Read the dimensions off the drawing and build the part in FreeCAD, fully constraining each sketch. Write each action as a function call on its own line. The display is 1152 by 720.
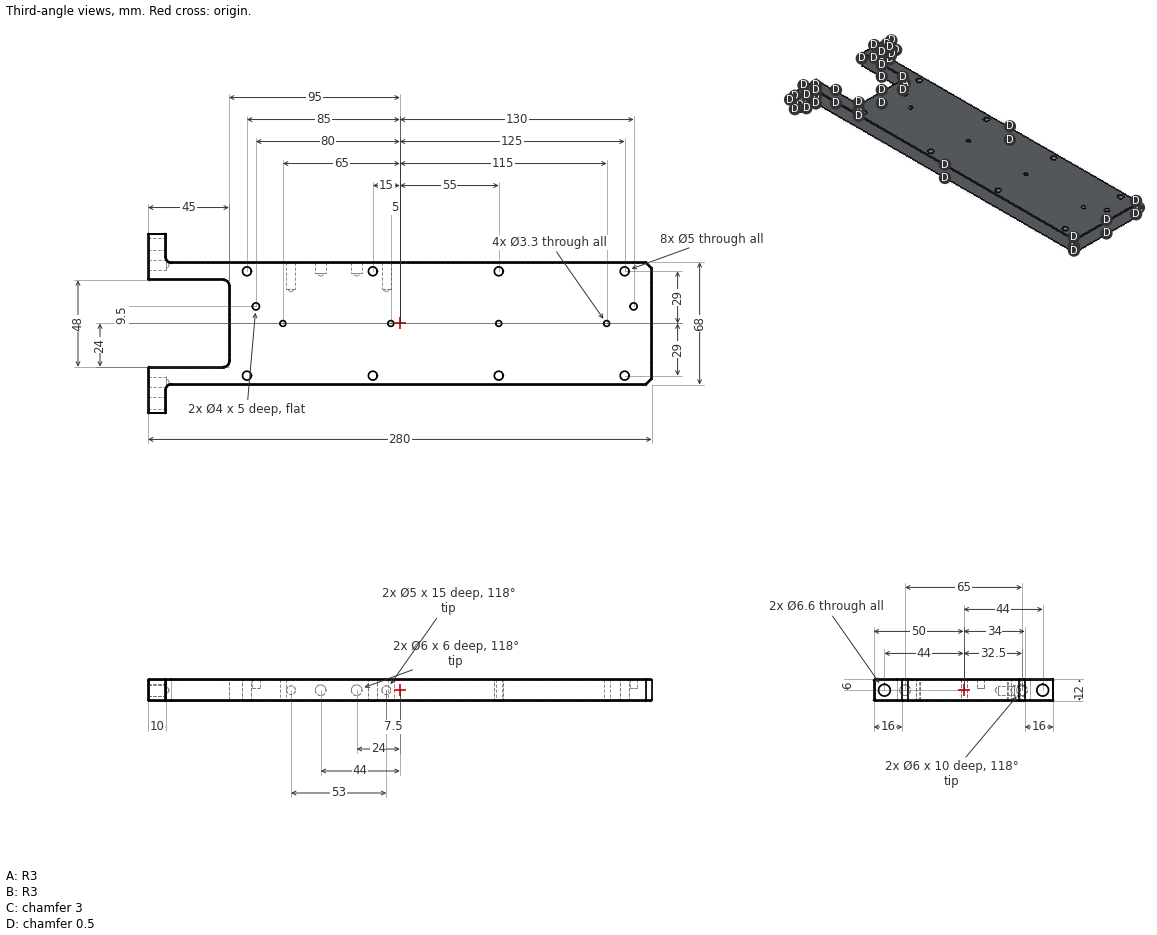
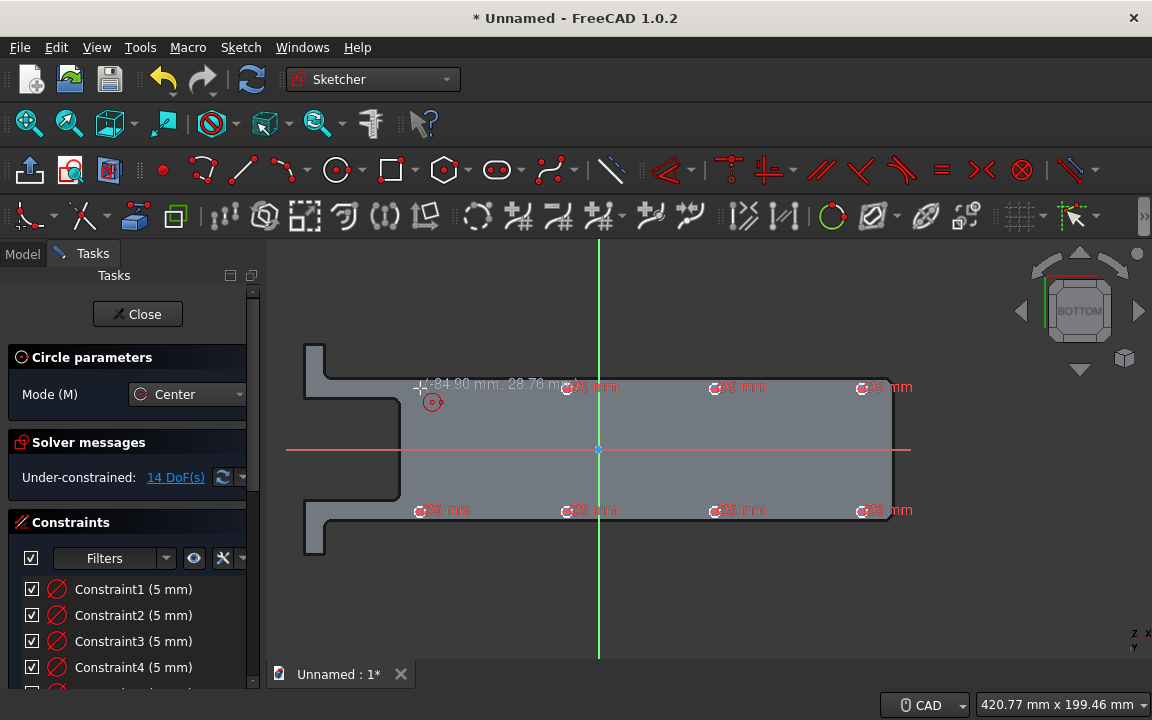
click(420, 388)
move(424, 385)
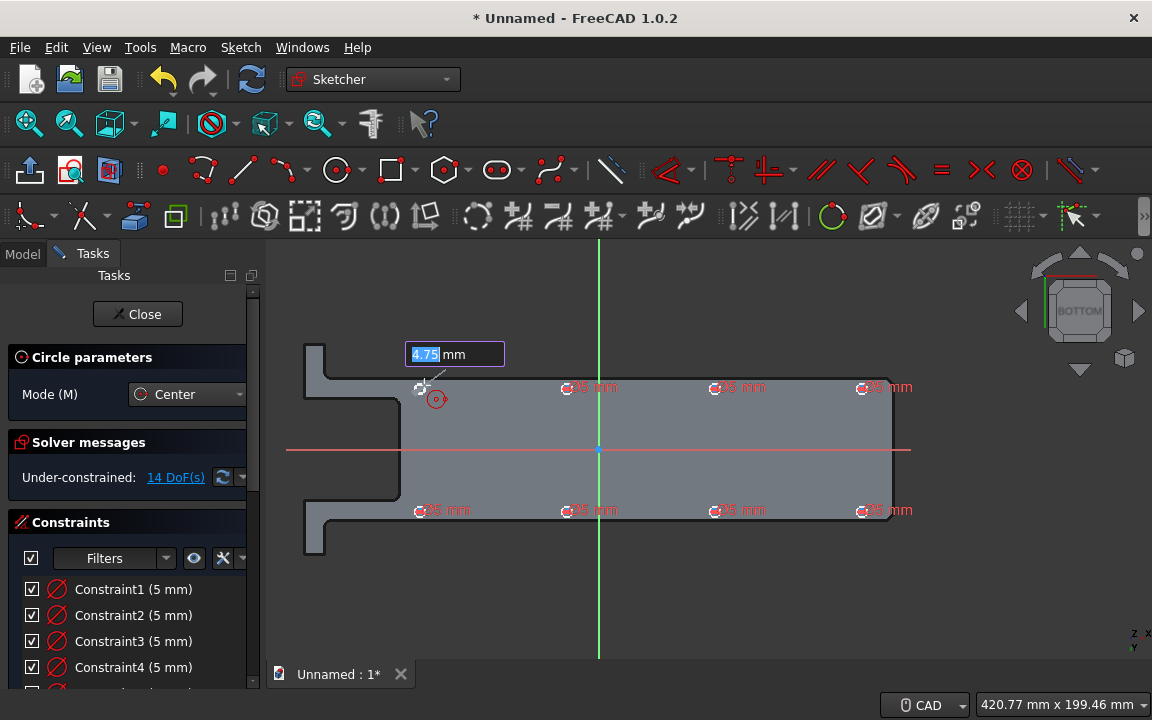
text(5)
key(Return)
key(Escape)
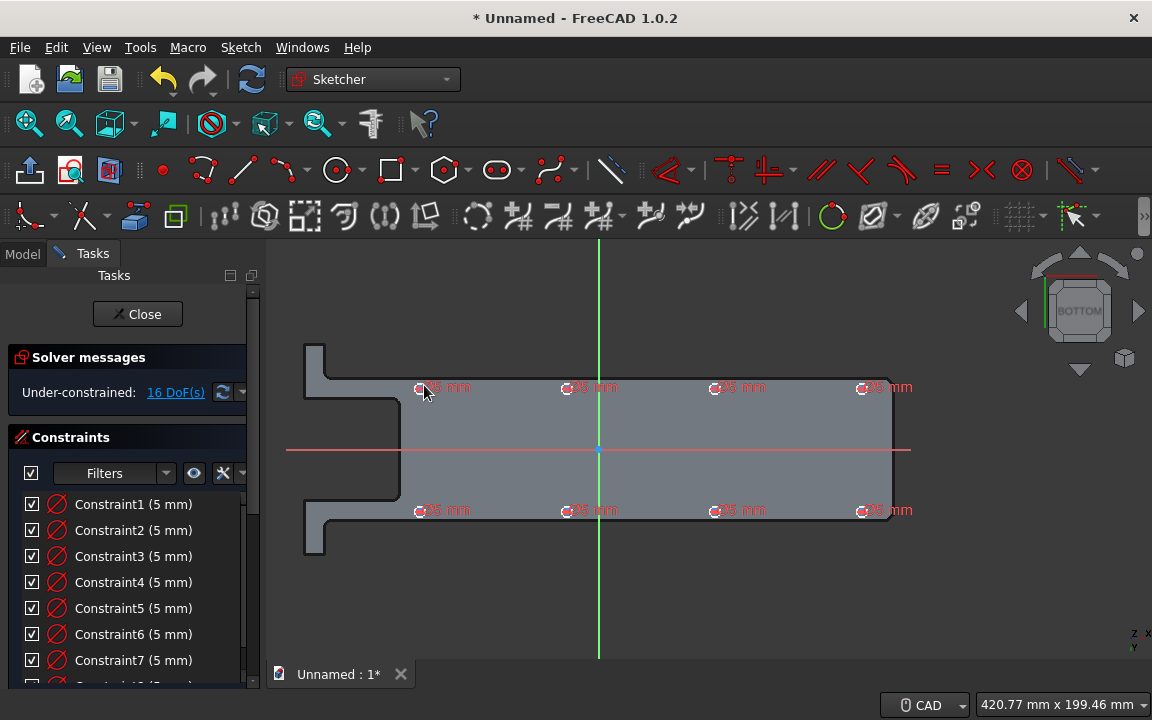
click(666, 170)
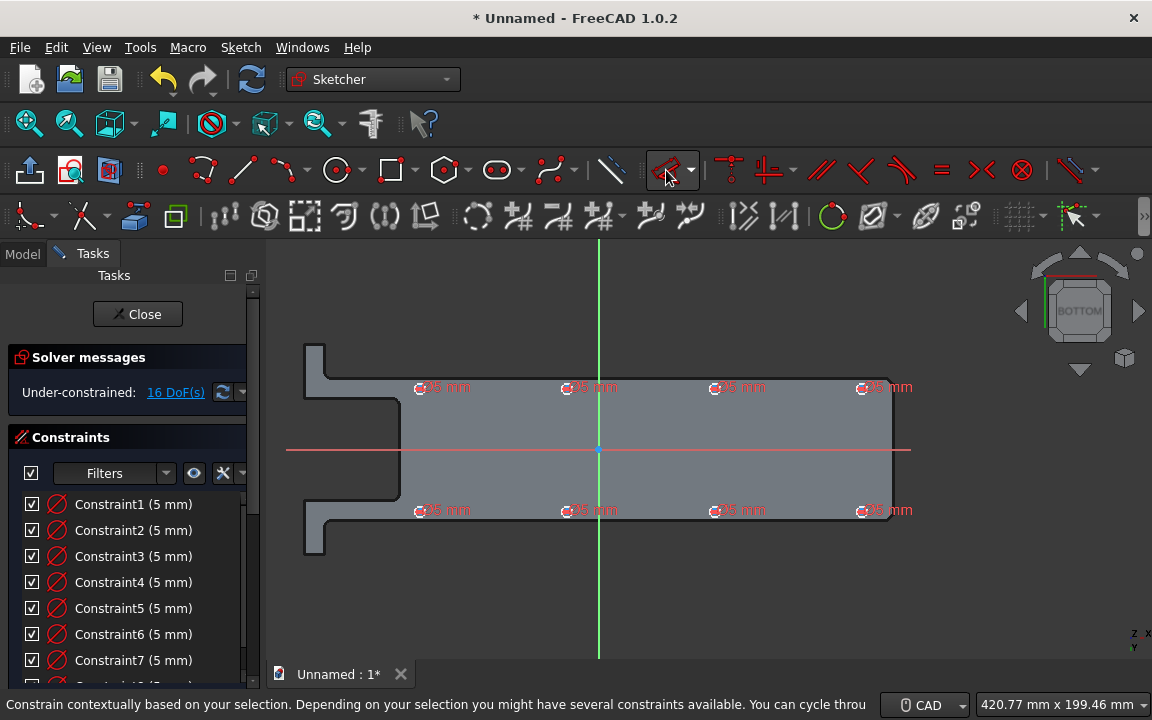
click(862, 512)
click(896, 481)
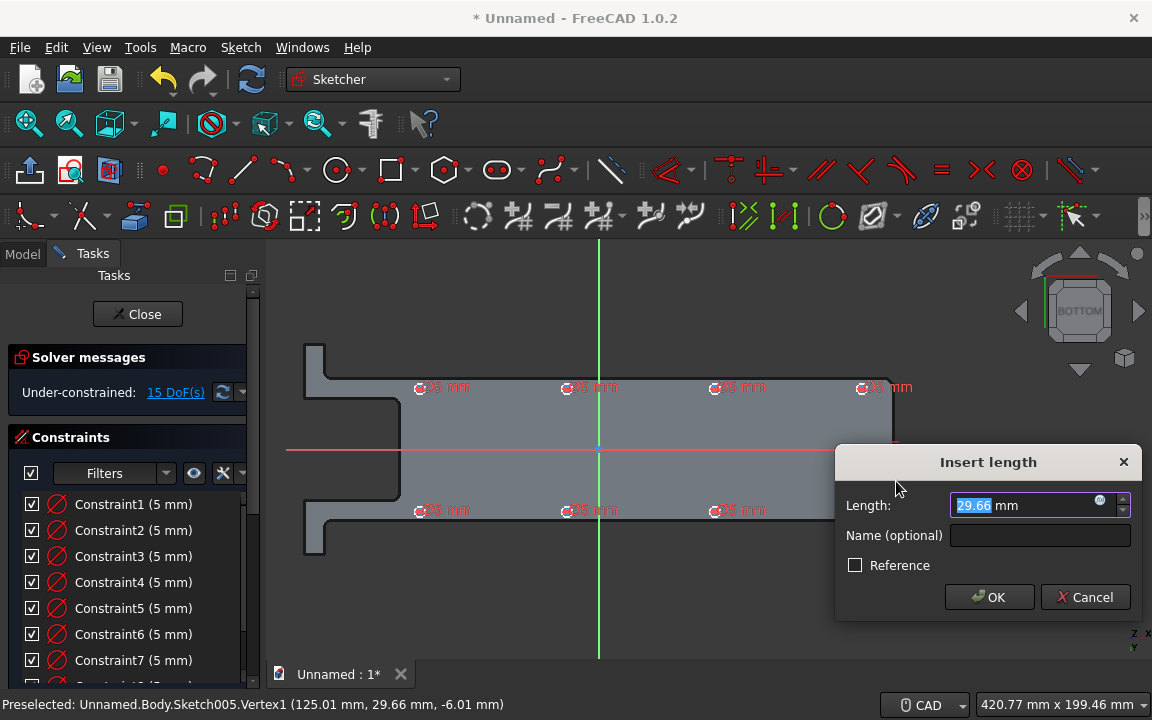
text(29)
key(Return)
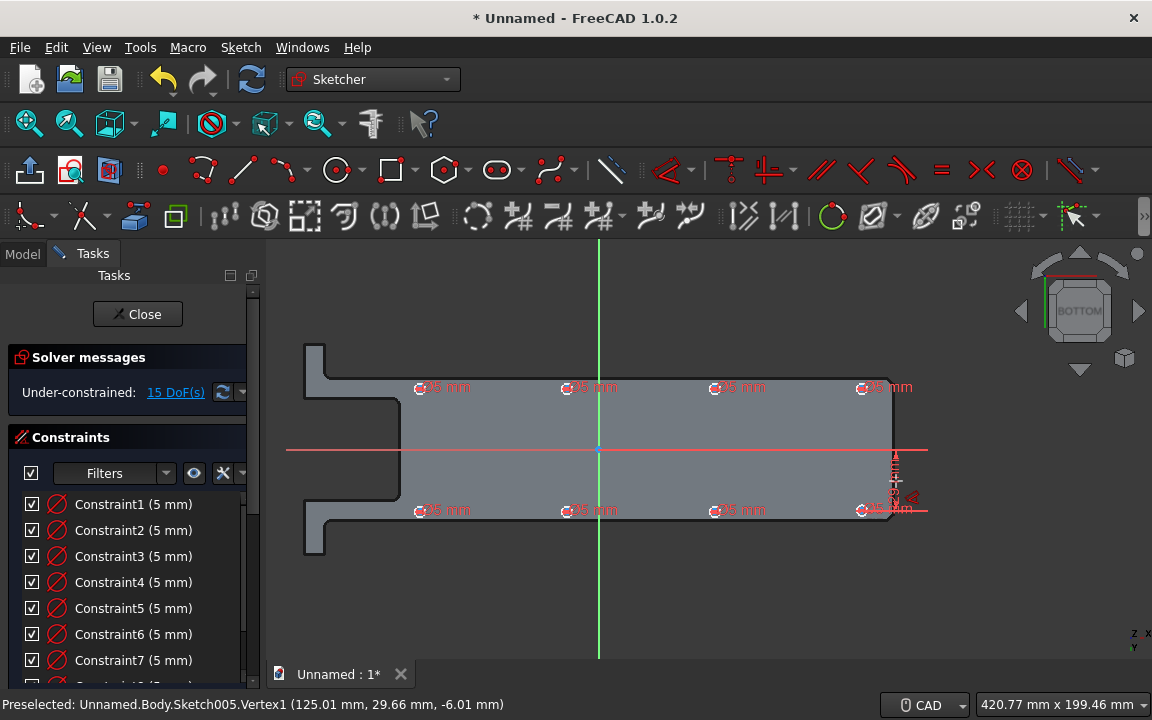
click(862, 389)
click(896, 419)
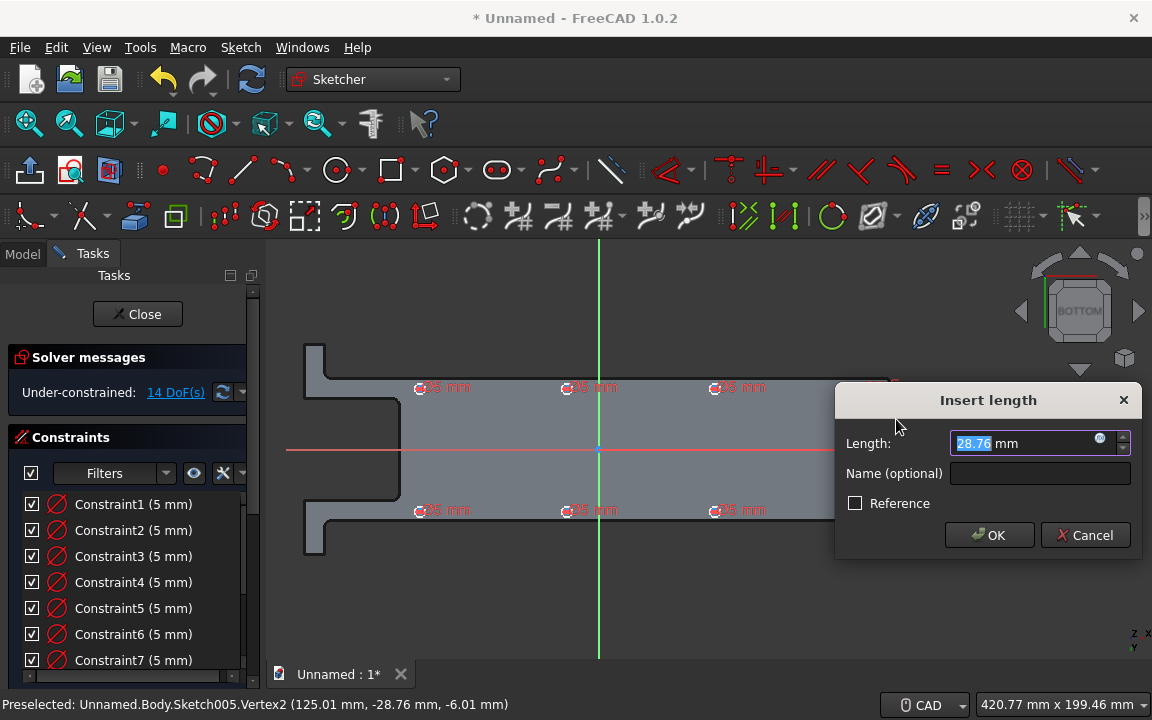
text(29)
key(Return)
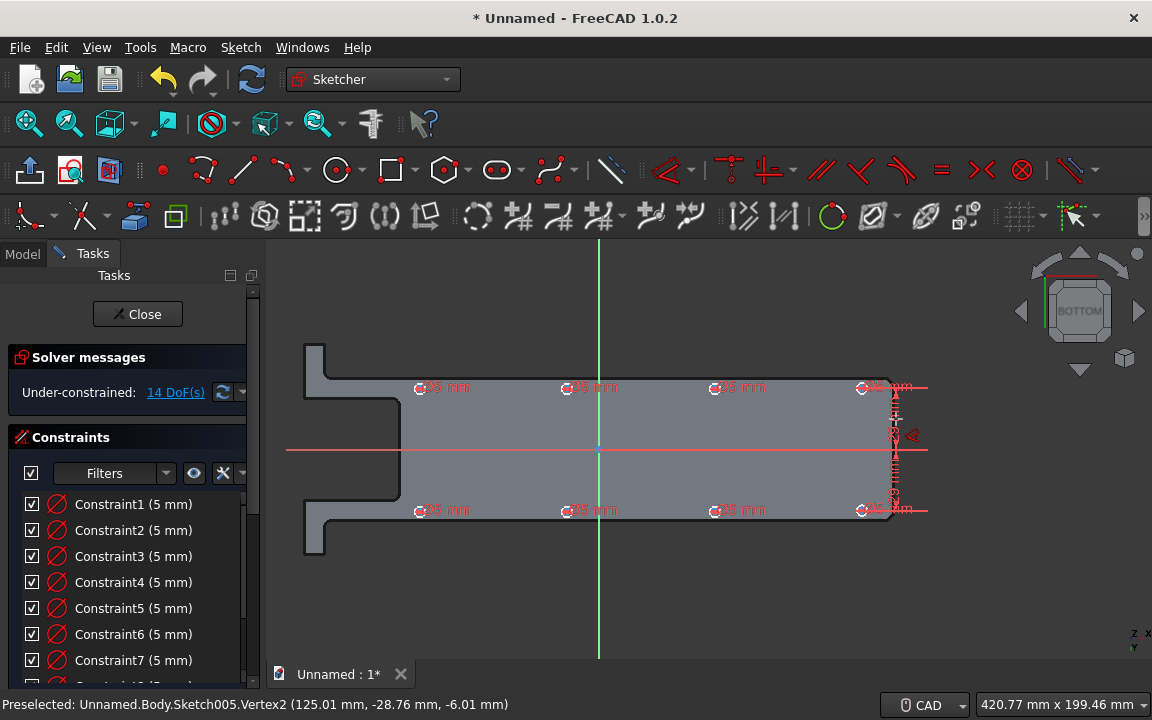
click(715, 512)
click(657, 546)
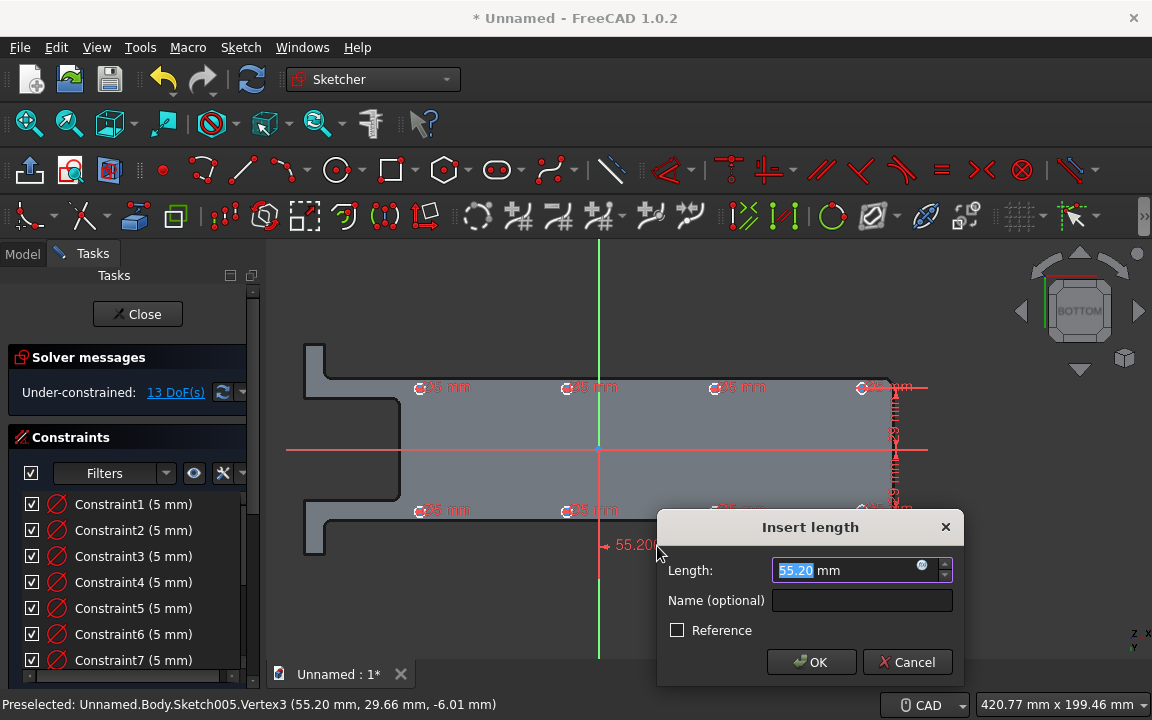
text(55)
key(Return)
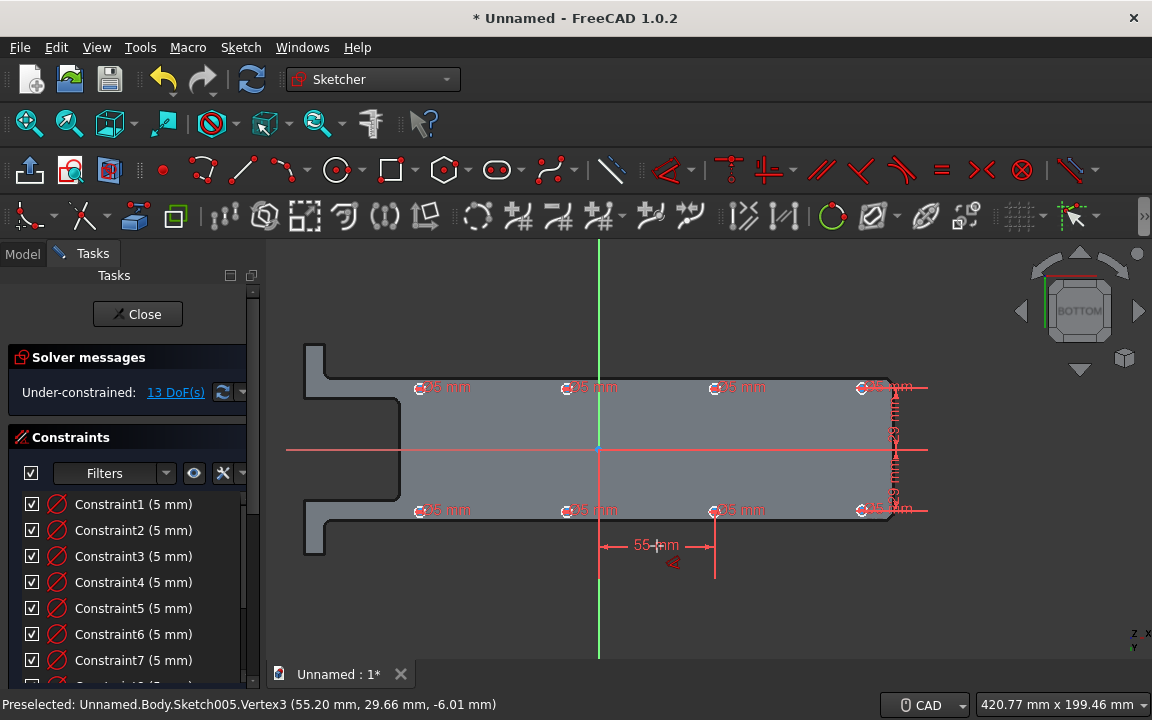
click(715, 512)
click(749, 481)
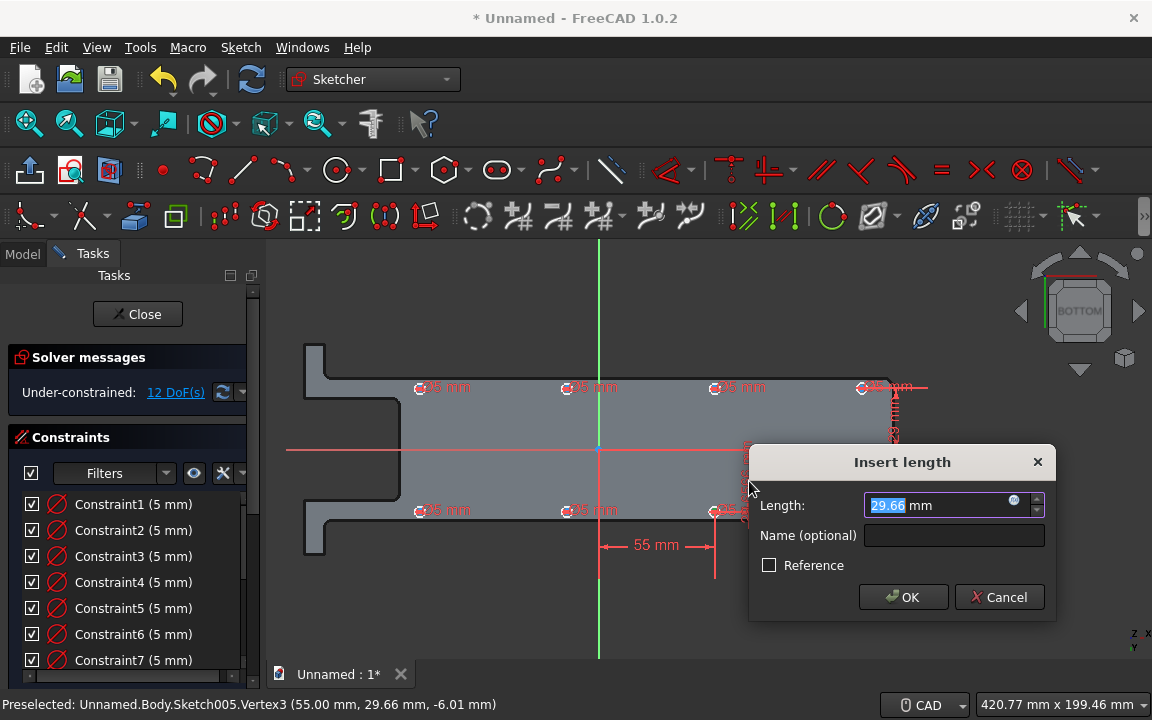
text(29)
key(Return)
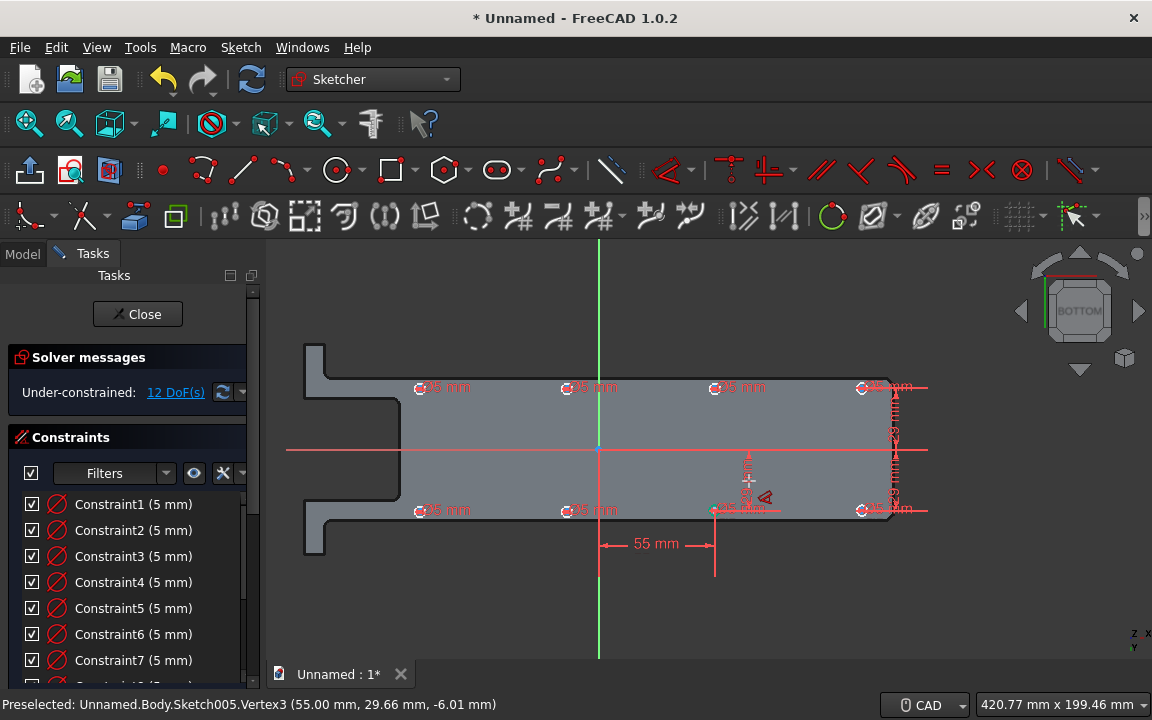
click(715, 389)
click(657, 355)